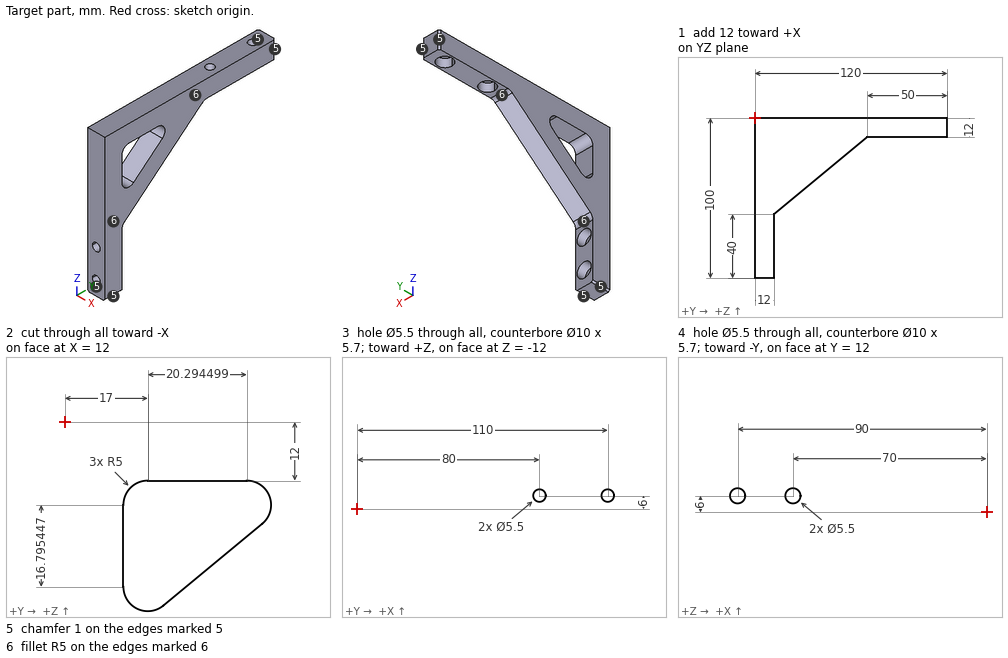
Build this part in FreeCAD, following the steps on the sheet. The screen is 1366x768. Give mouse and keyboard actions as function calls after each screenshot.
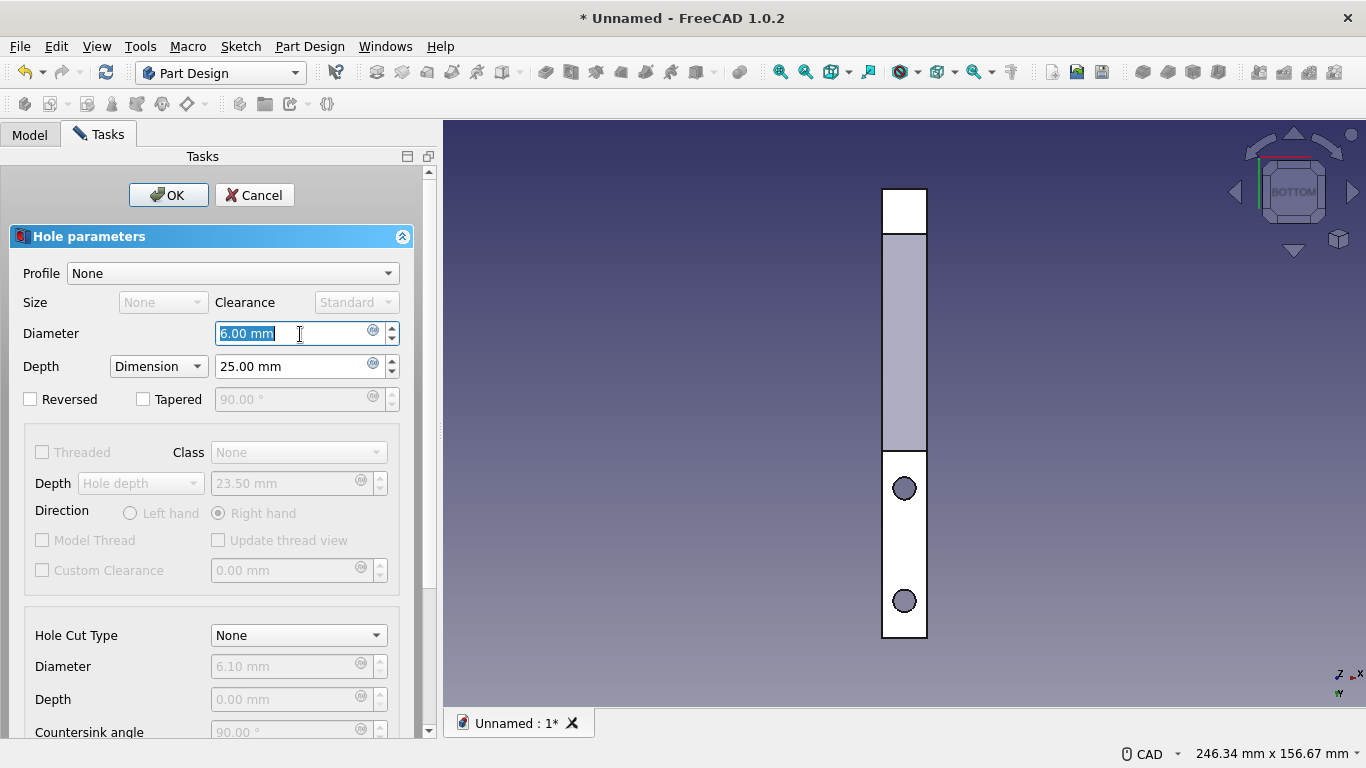
text(5.5)
key(Tab)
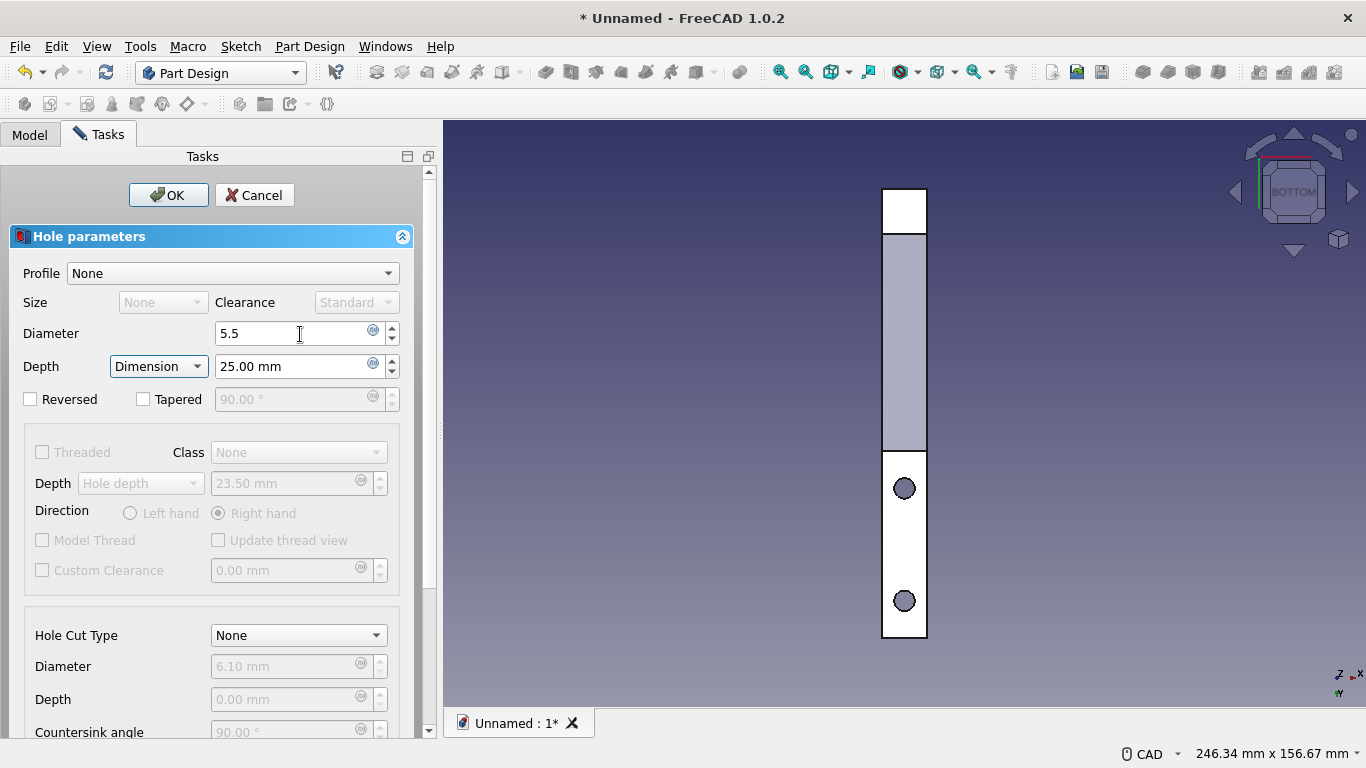
click(160, 366)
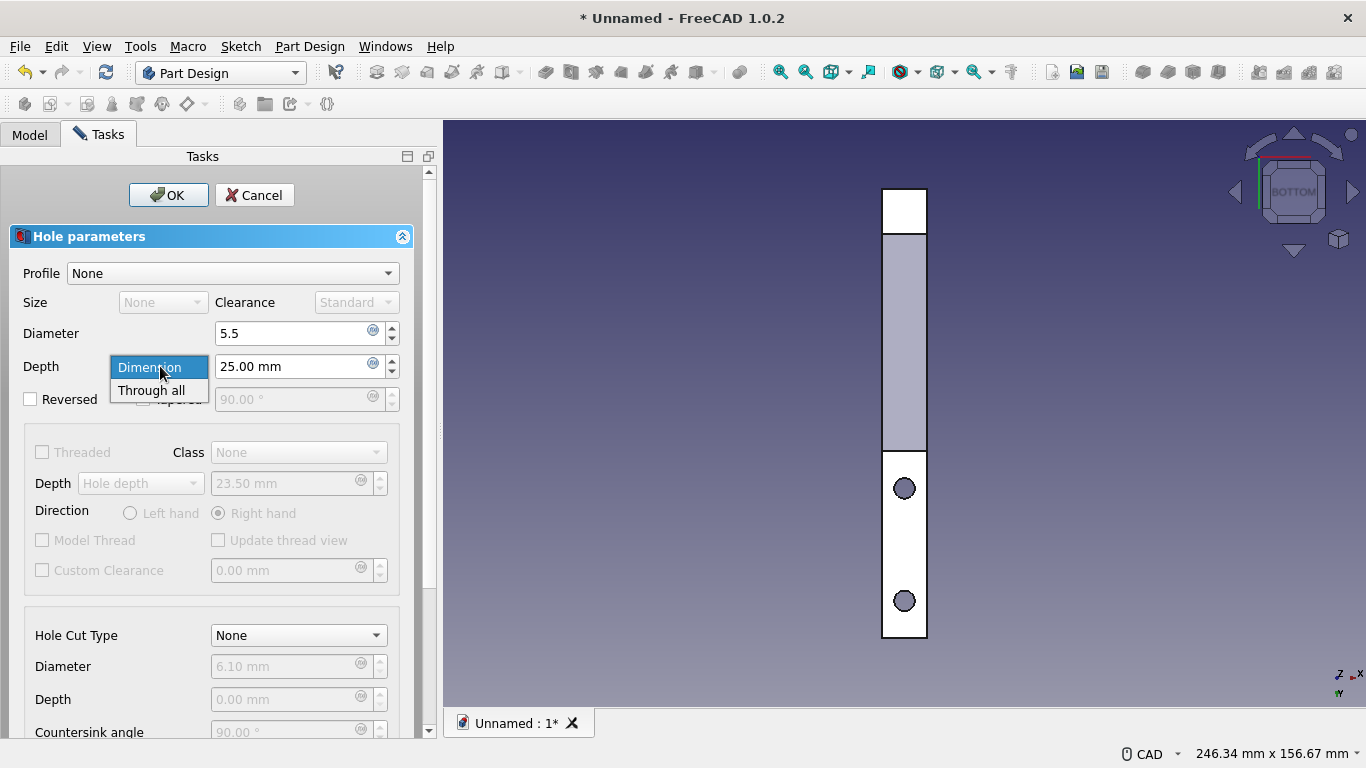
click(158, 390)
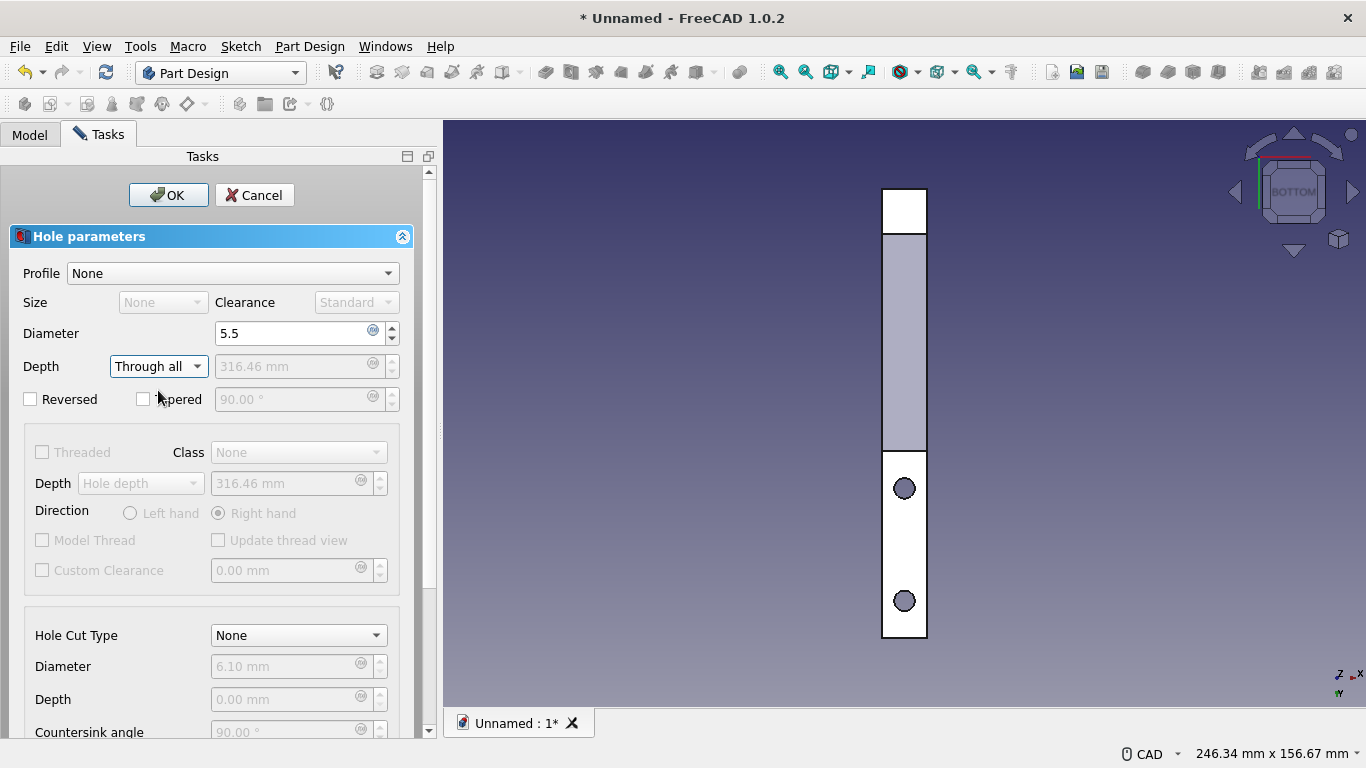
click(300, 636)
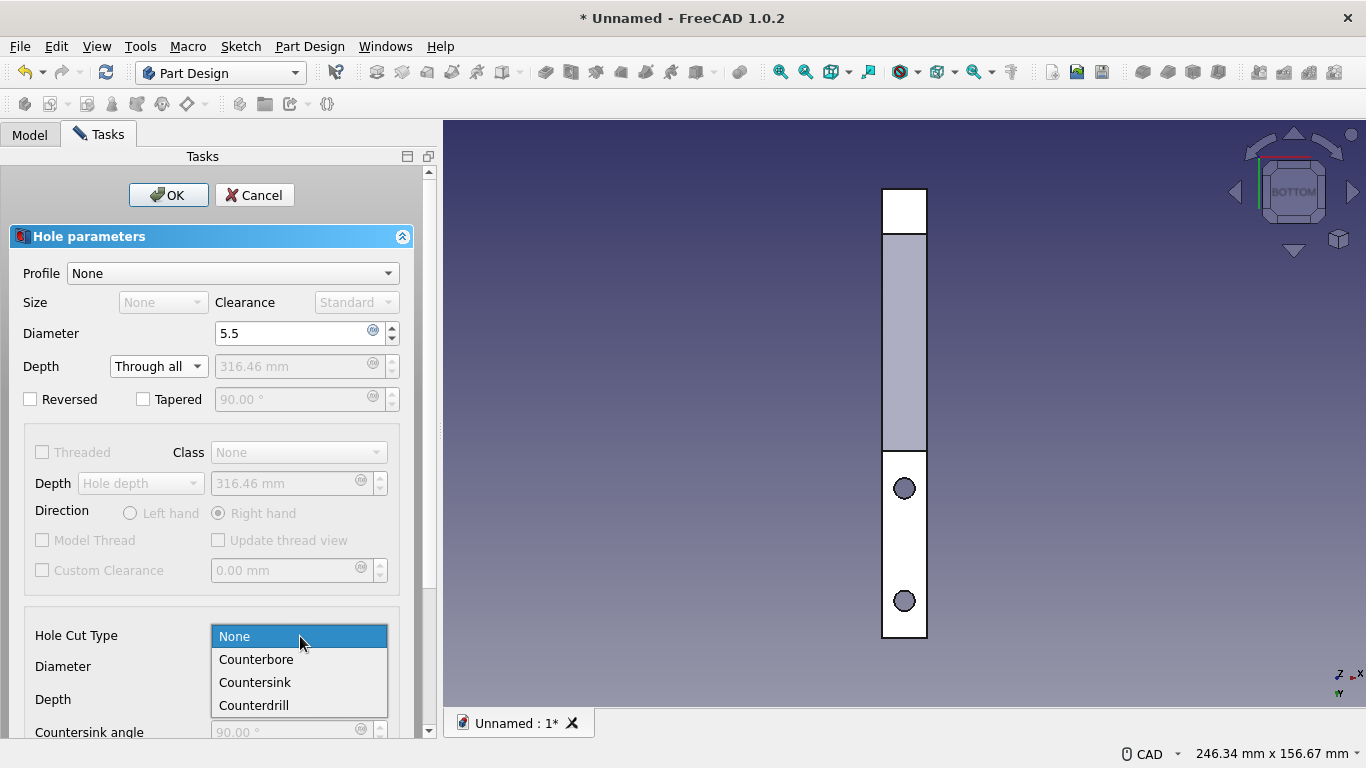
click(298, 660)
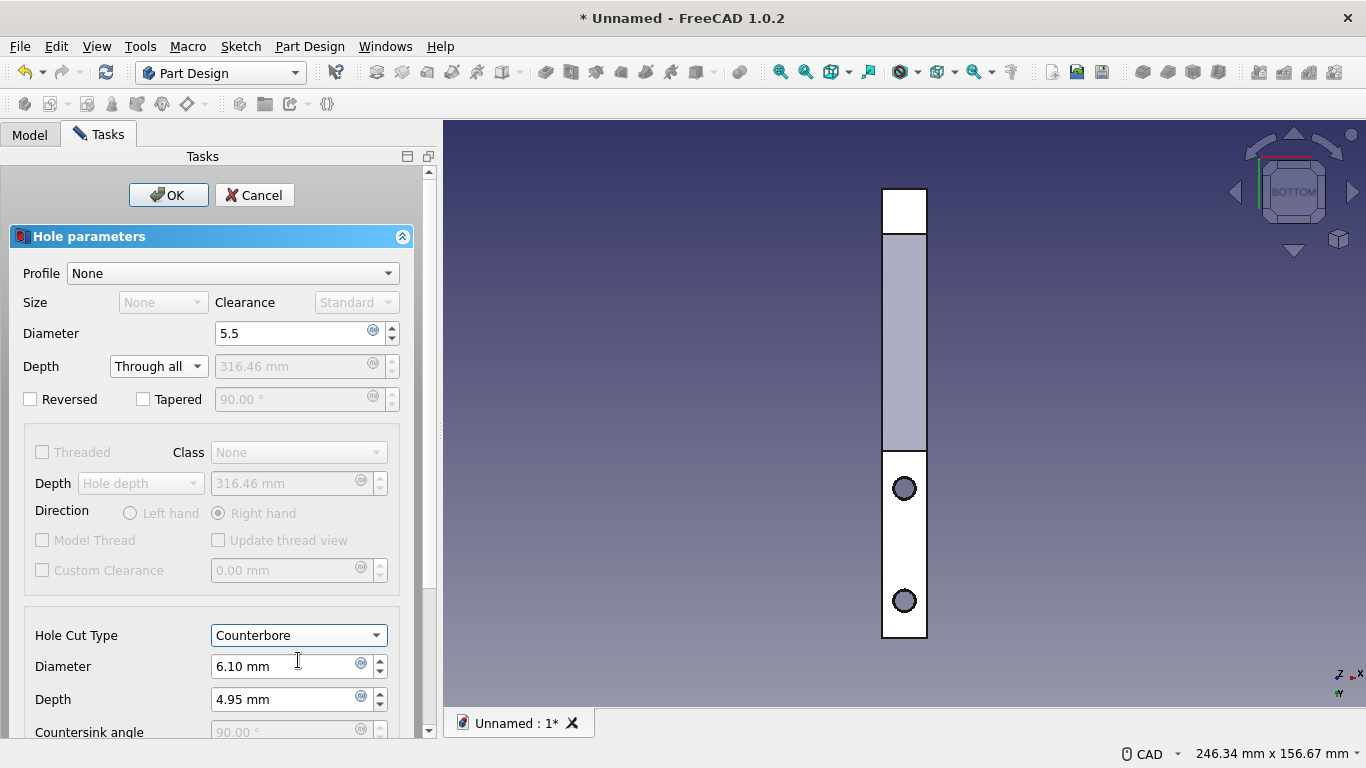
triple_click(292, 666)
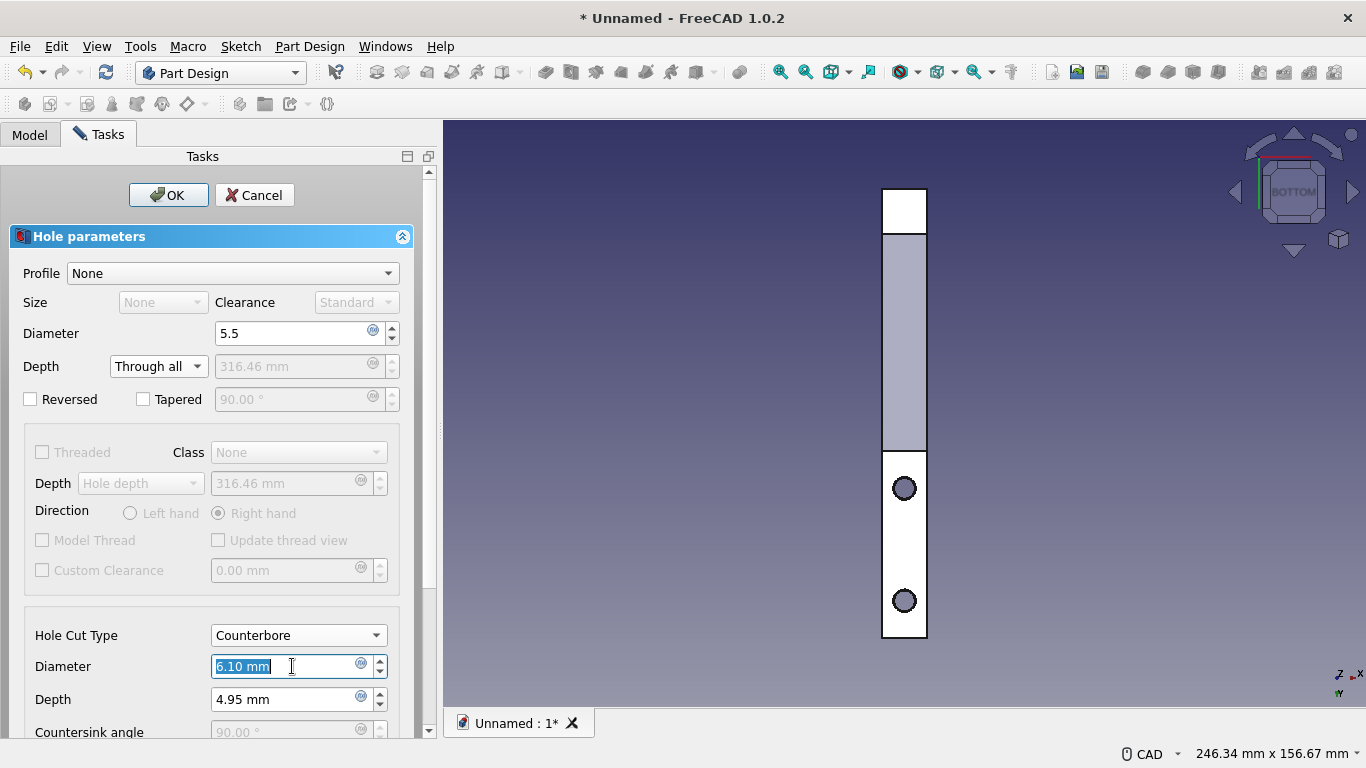
text(10)
key(Tab)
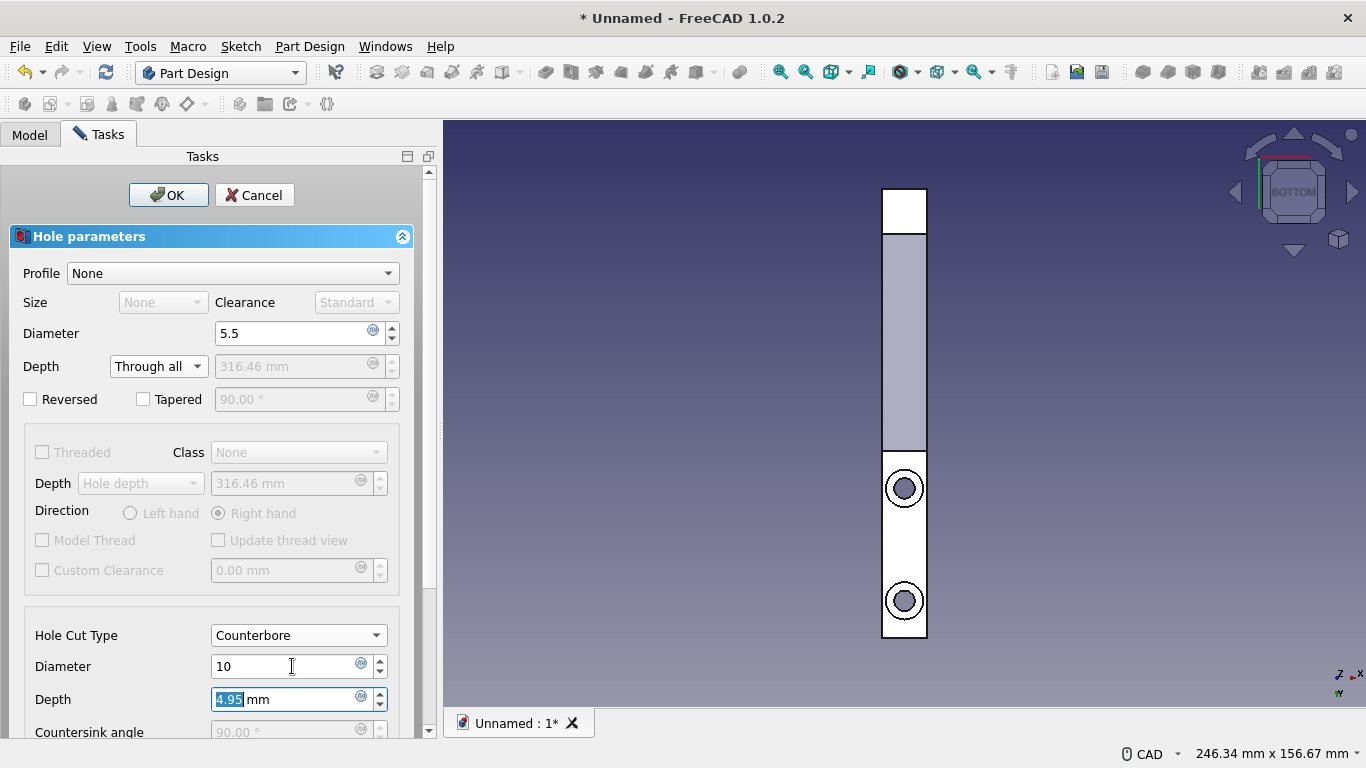
text(5.7)
key(Tab)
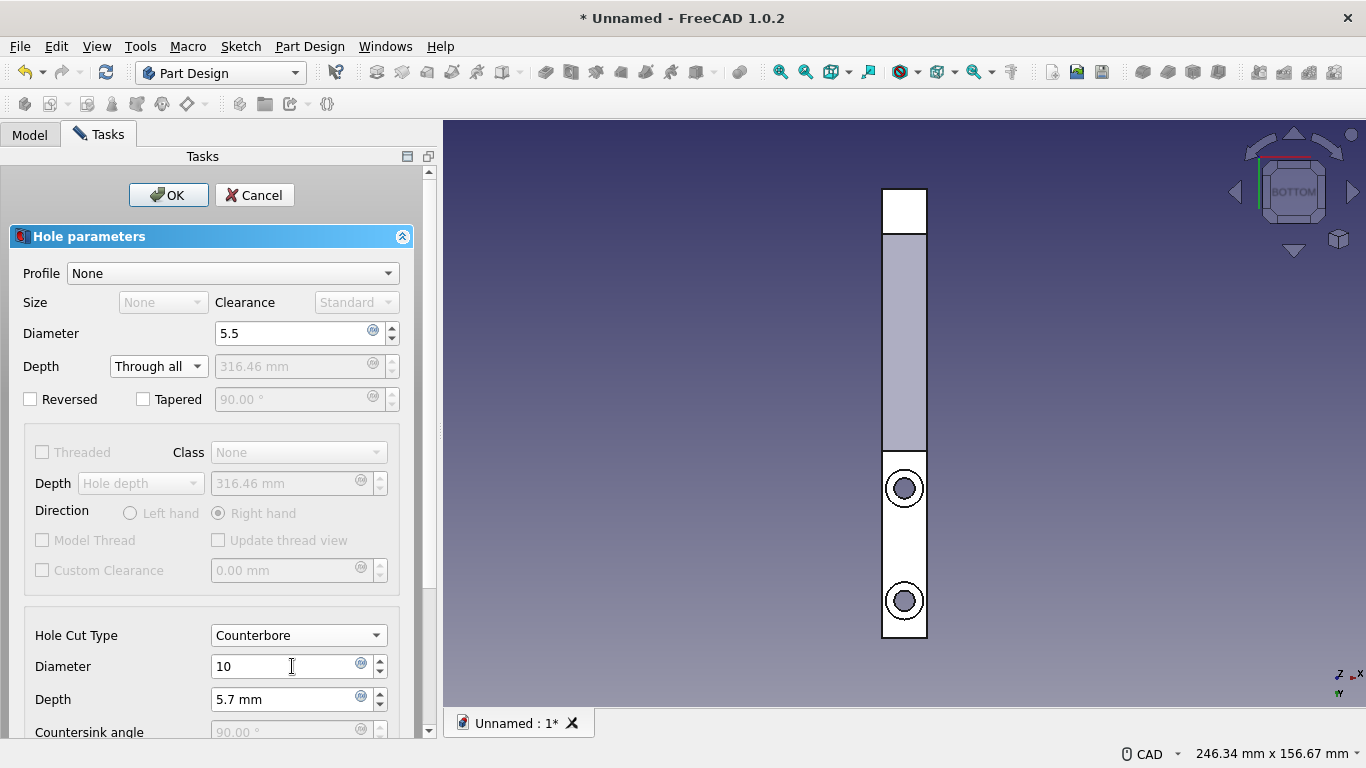
click(169, 195)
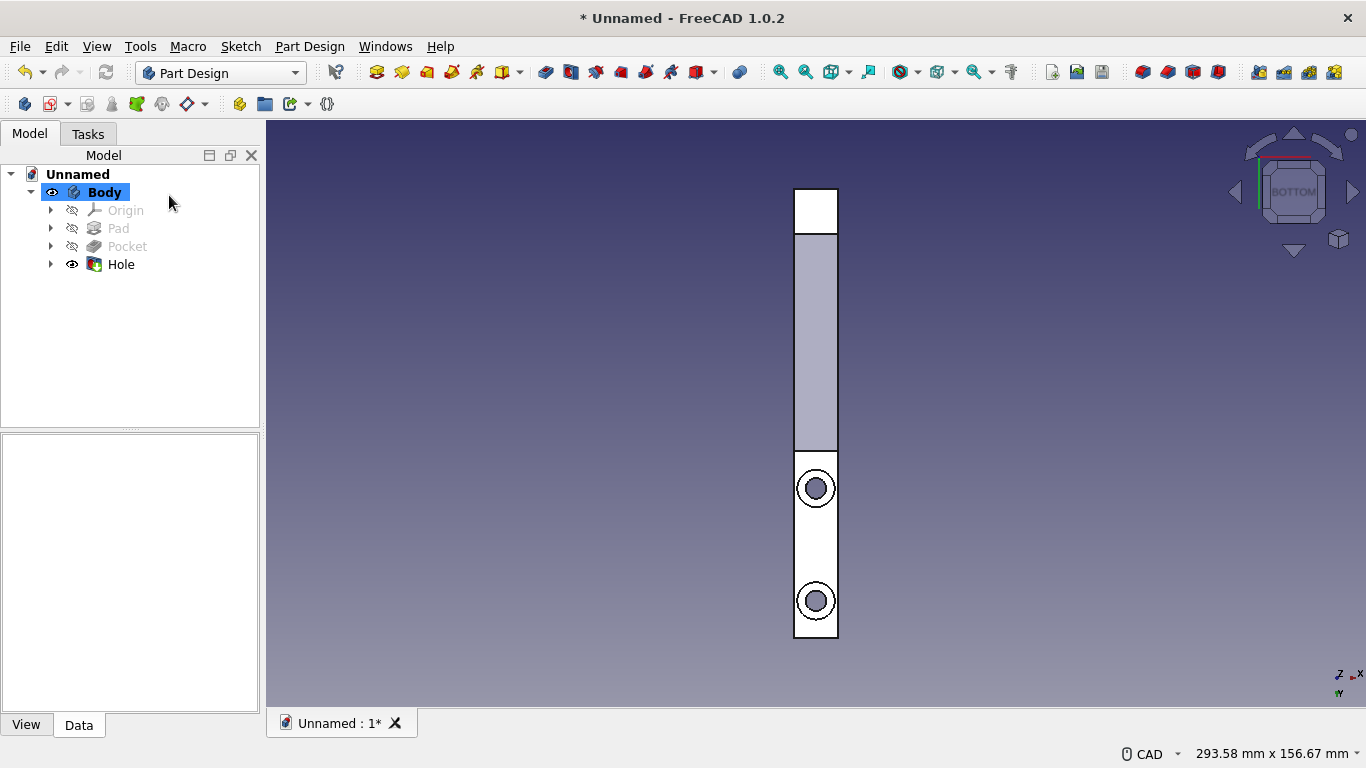
key(4)